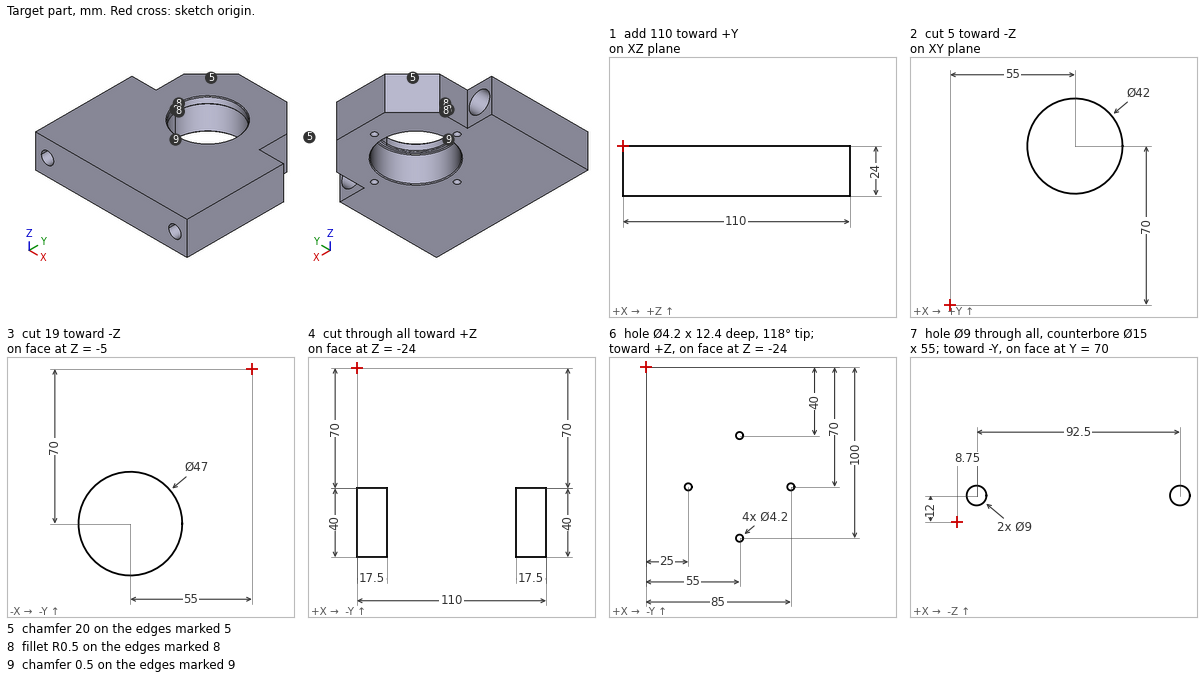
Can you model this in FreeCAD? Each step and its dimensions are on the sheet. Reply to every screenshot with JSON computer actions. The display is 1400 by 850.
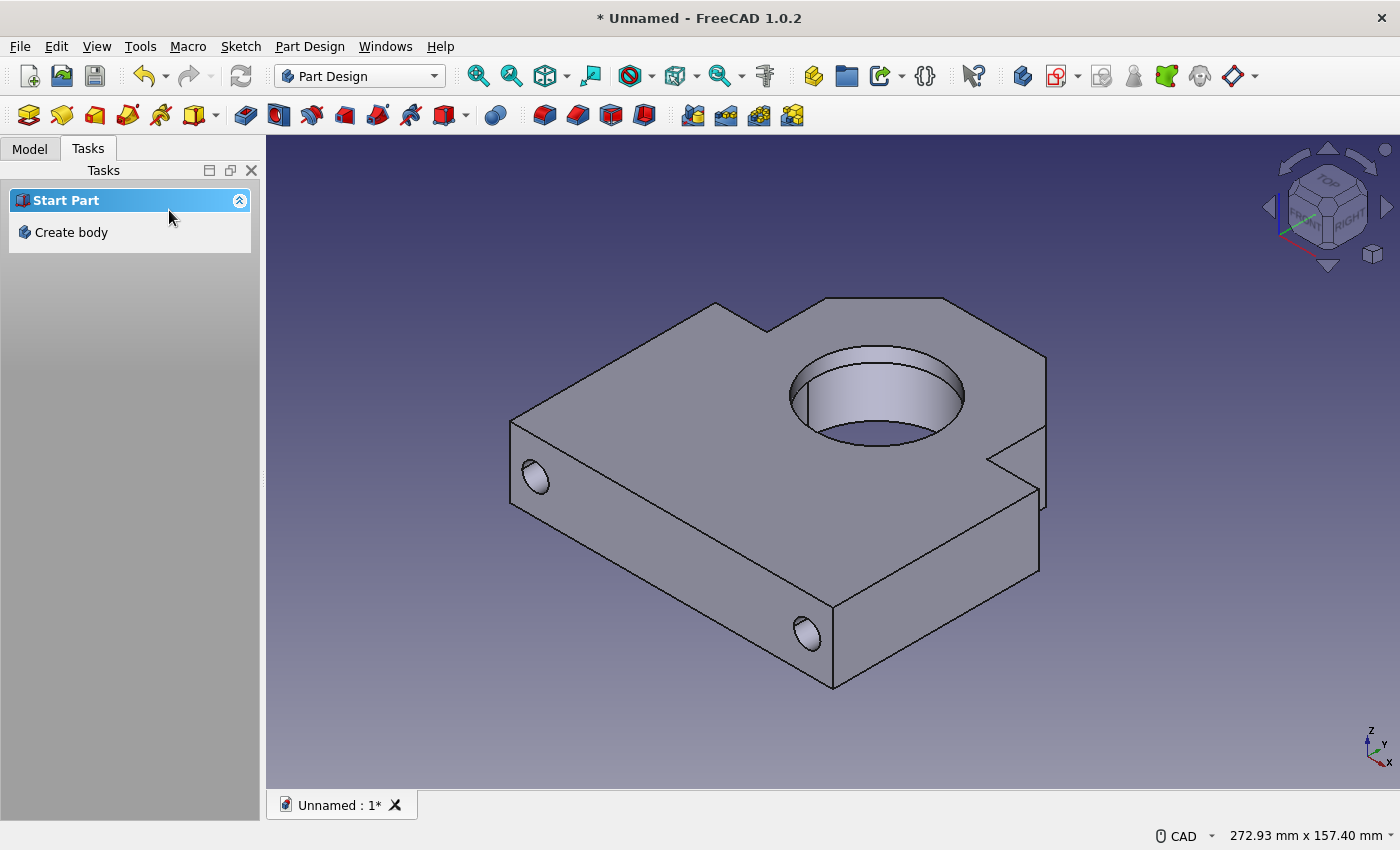
{"action": "left_click", "coordinate": [815, 359]}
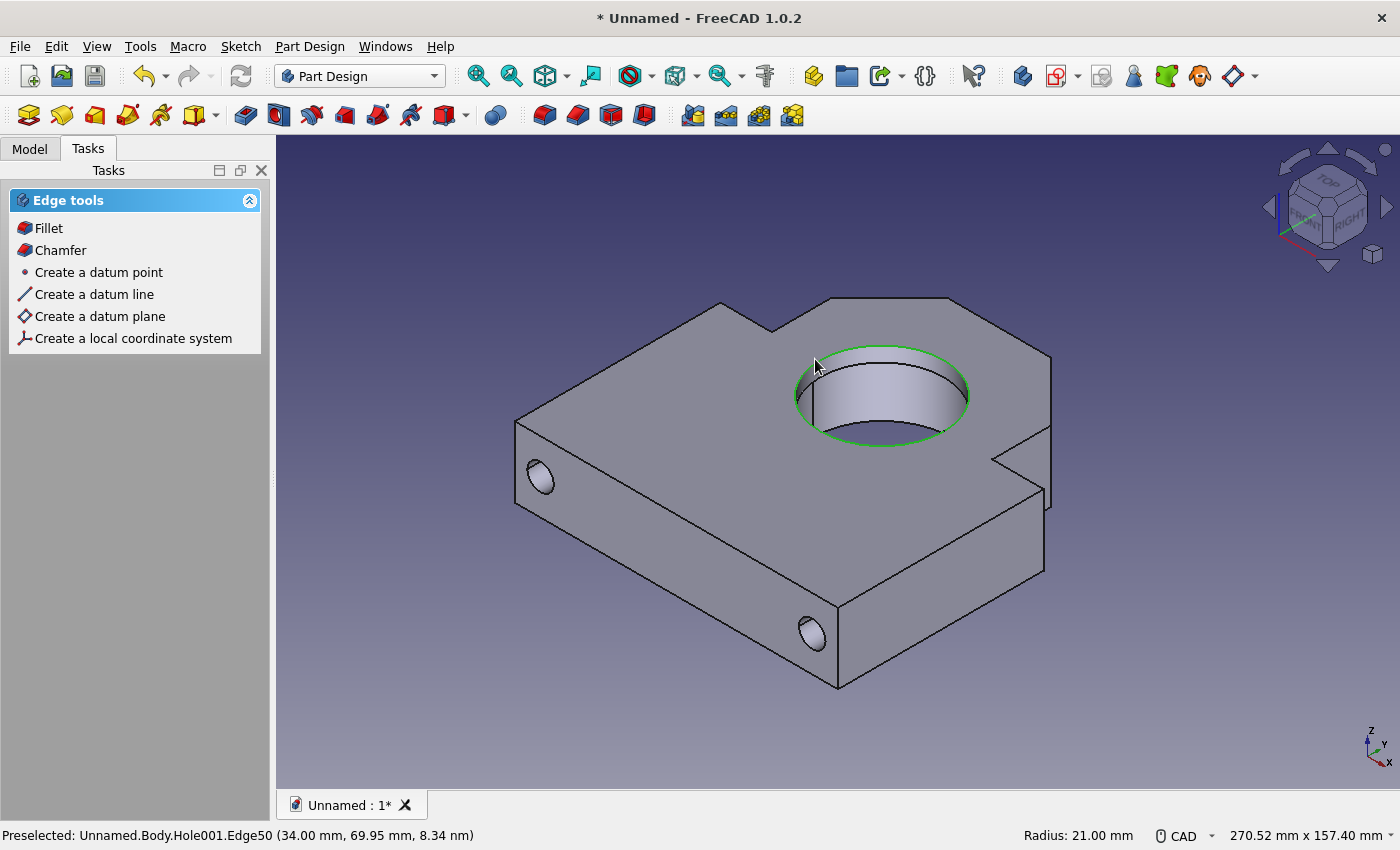
{"action": "key", "text": "2"}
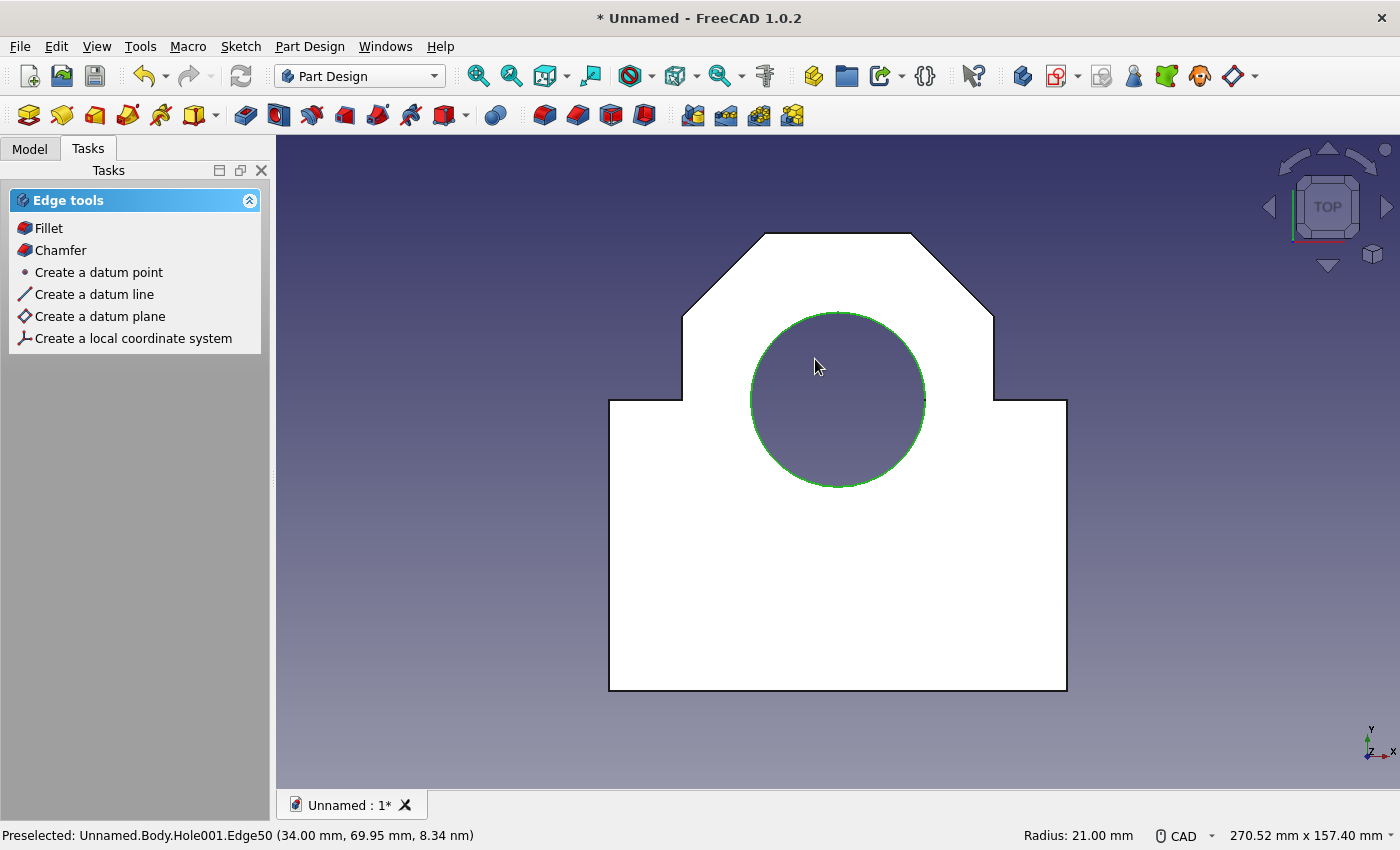
{"action": "key", "text": "1"}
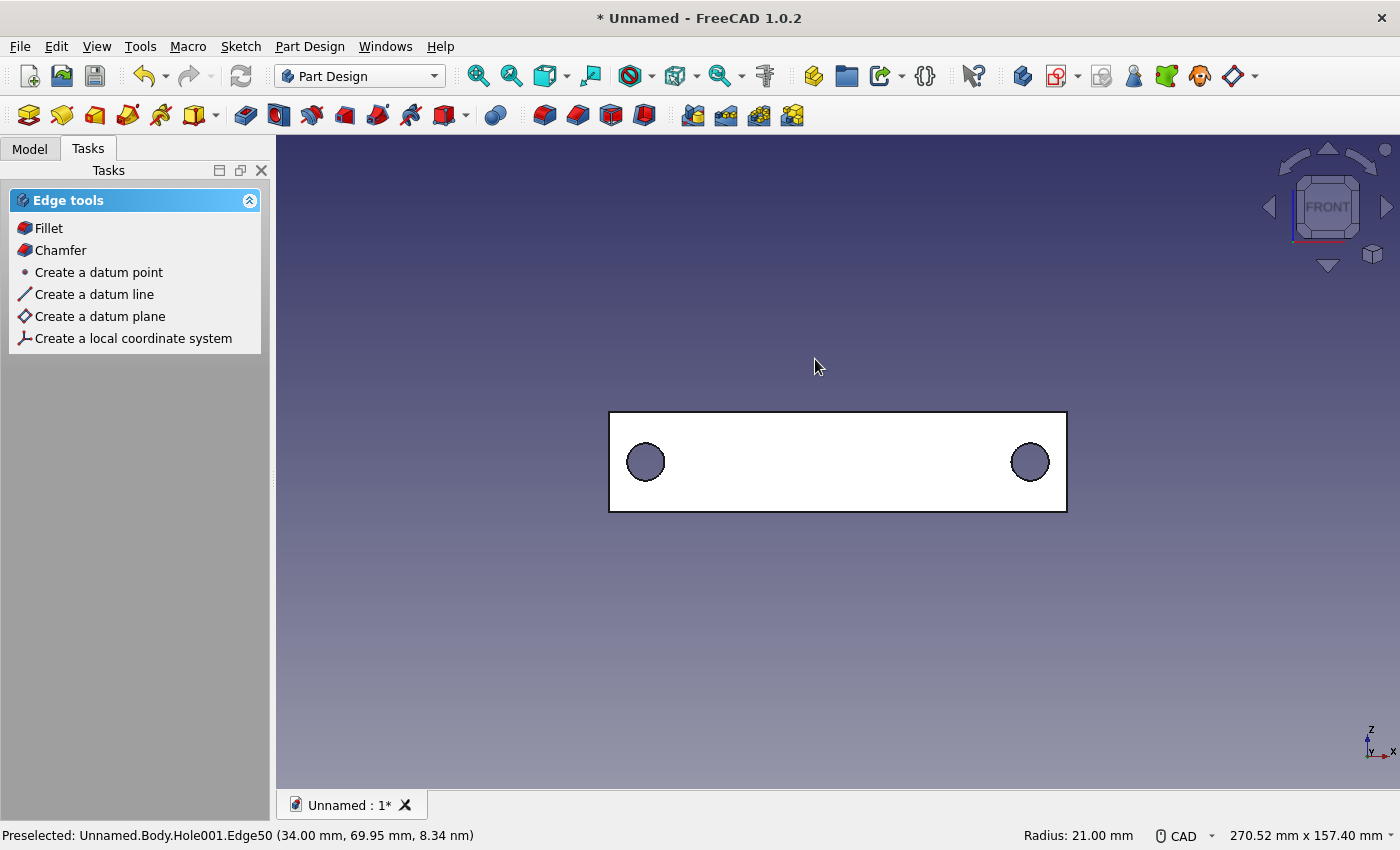
{"action": "key", "text": "v f"}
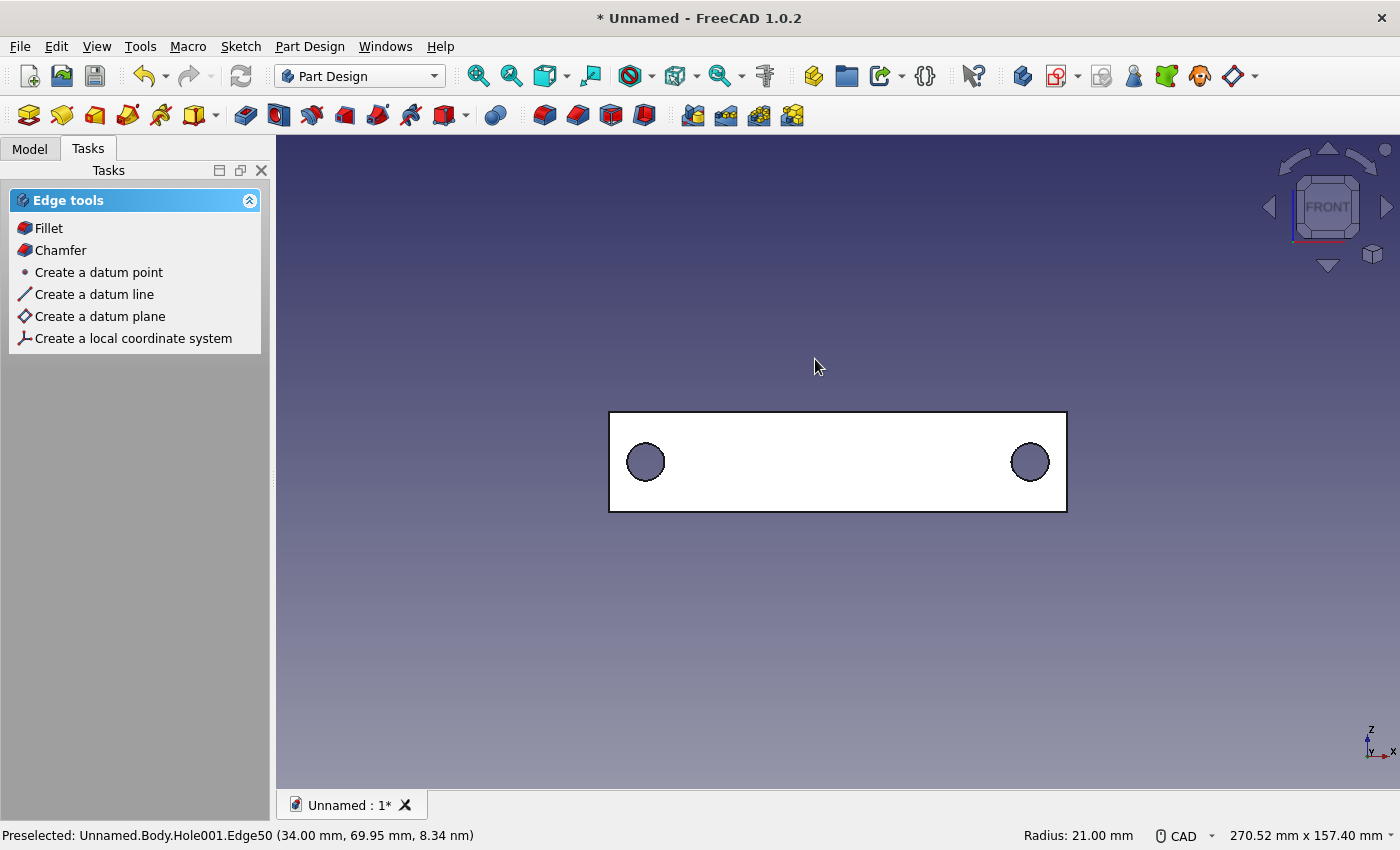
{"action": "key", "text": "3"}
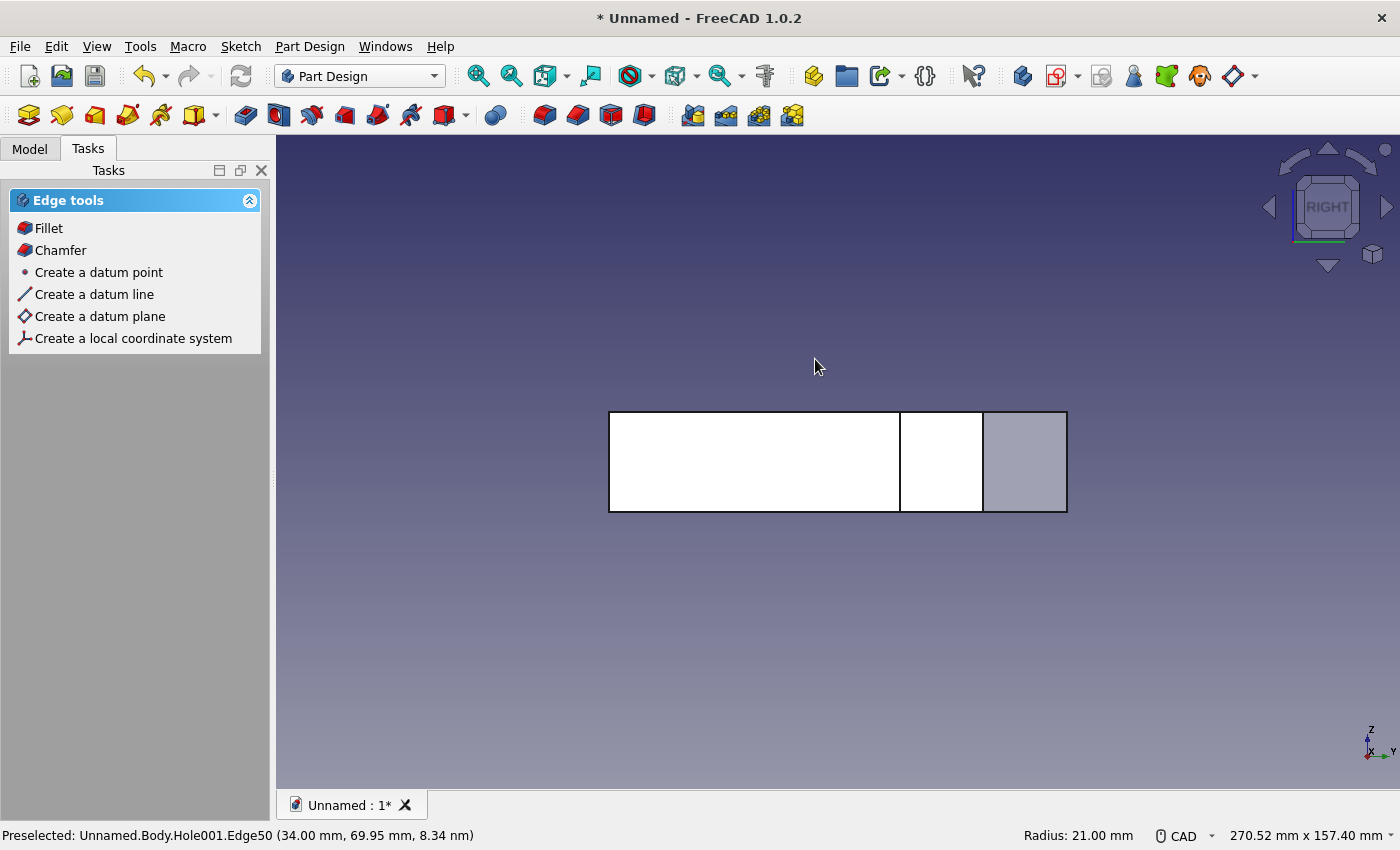
{"action": "left_click", "coordinate": [479, 76]}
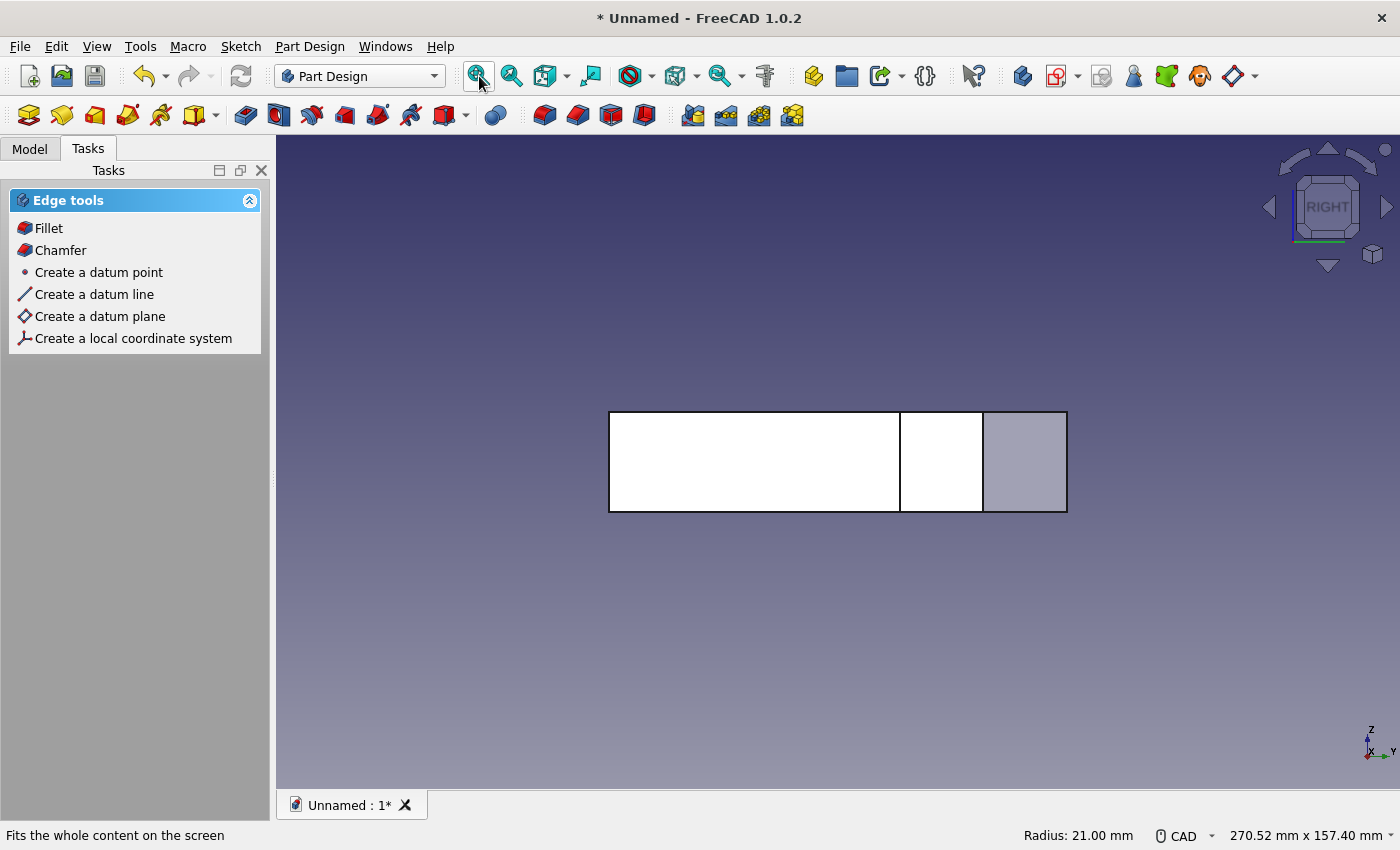
{"action": "key", "text": "5"}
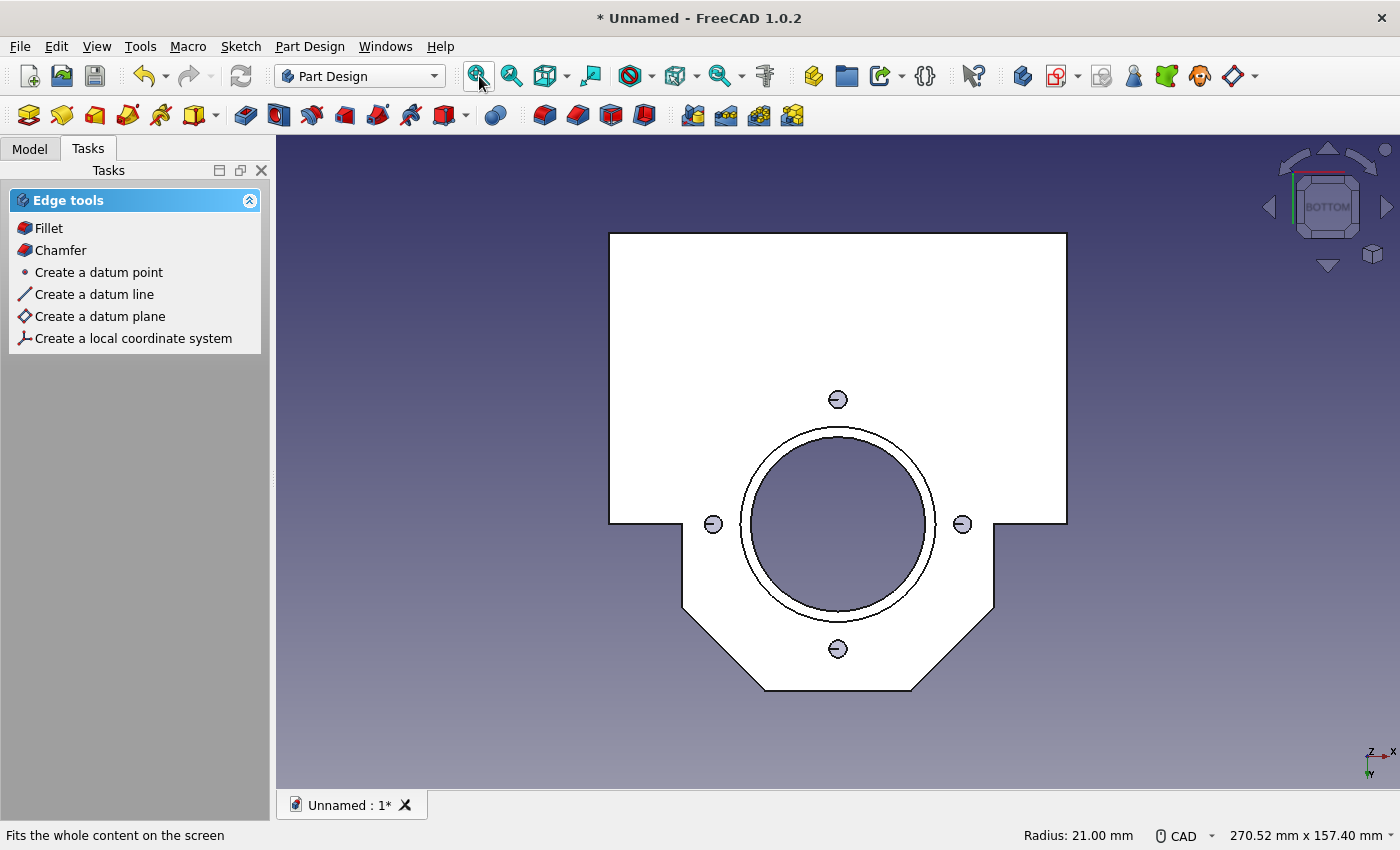
{"action": "left_click", "coordinate": [767, 575], "text": "ctrl"}